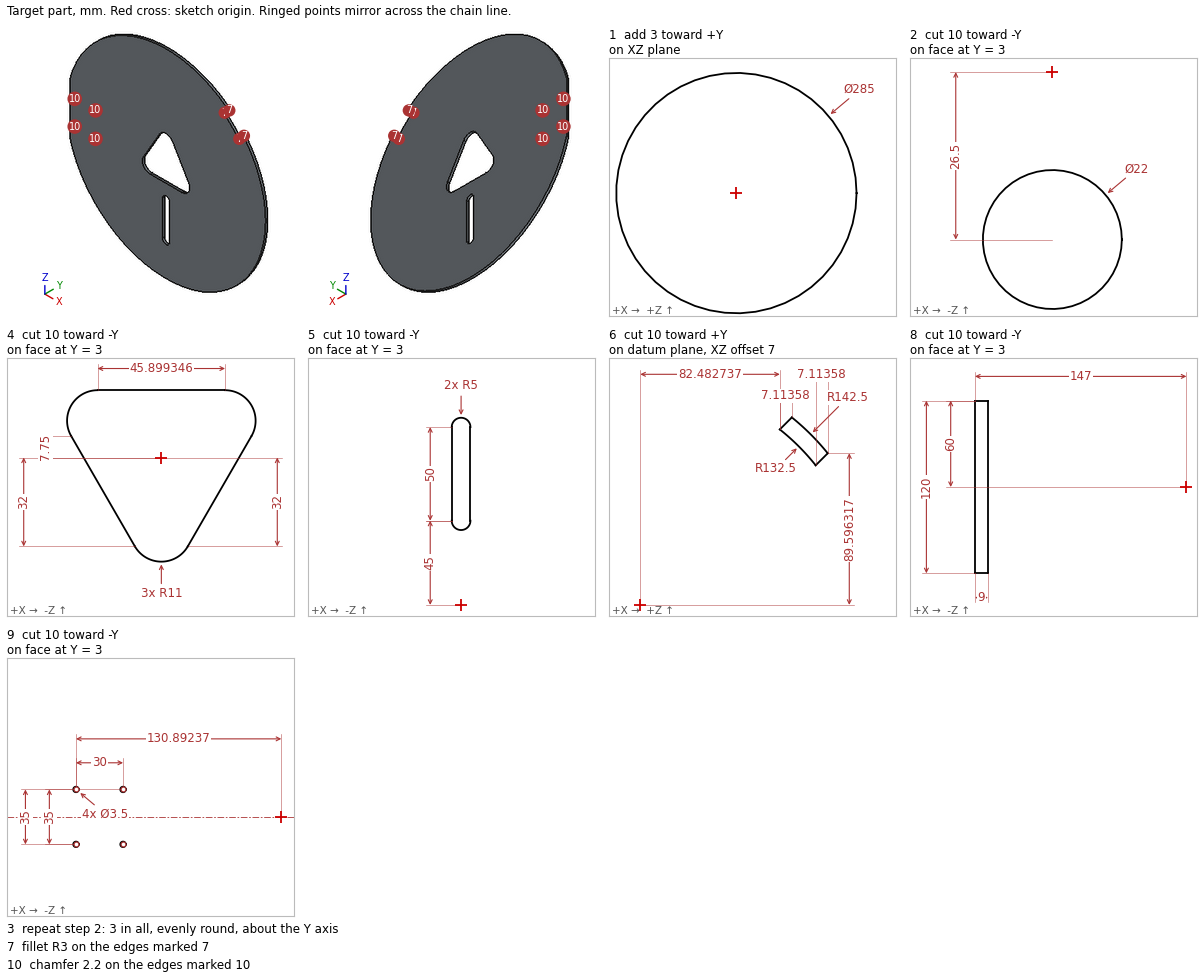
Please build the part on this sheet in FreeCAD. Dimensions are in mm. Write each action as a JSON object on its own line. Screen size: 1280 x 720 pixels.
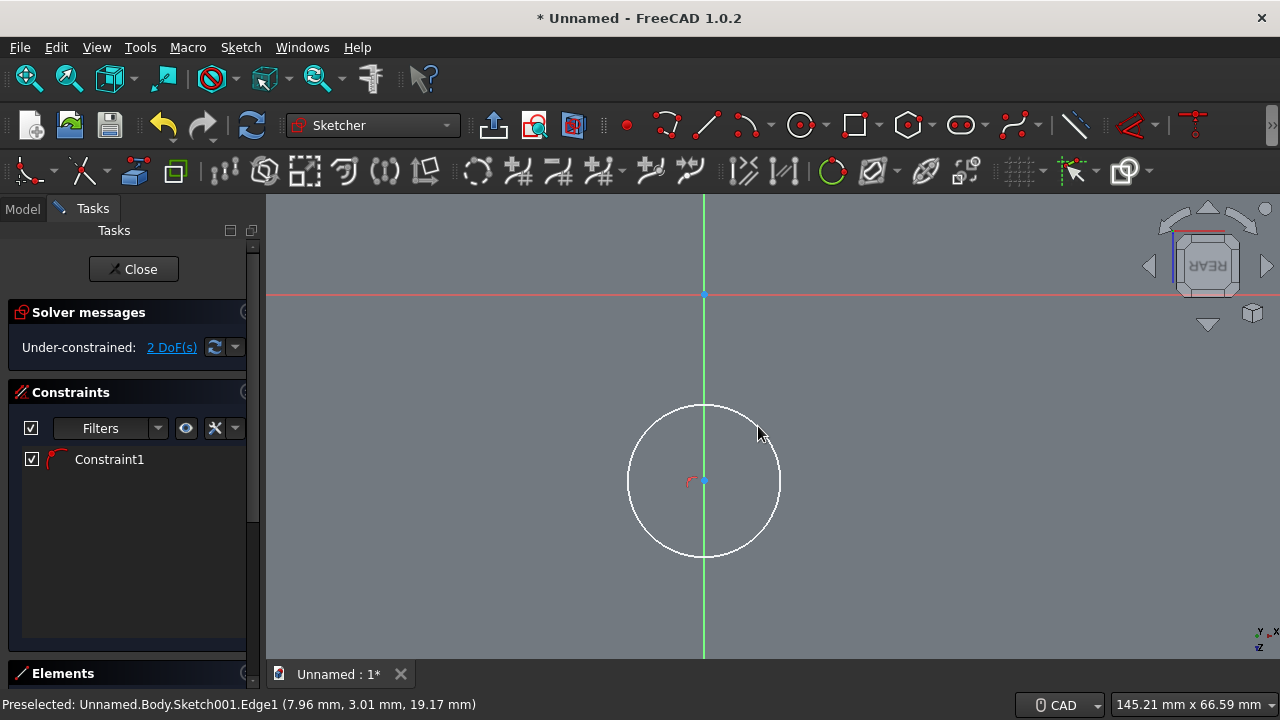
{"action": "left_click", "coordinate": [758, 427]}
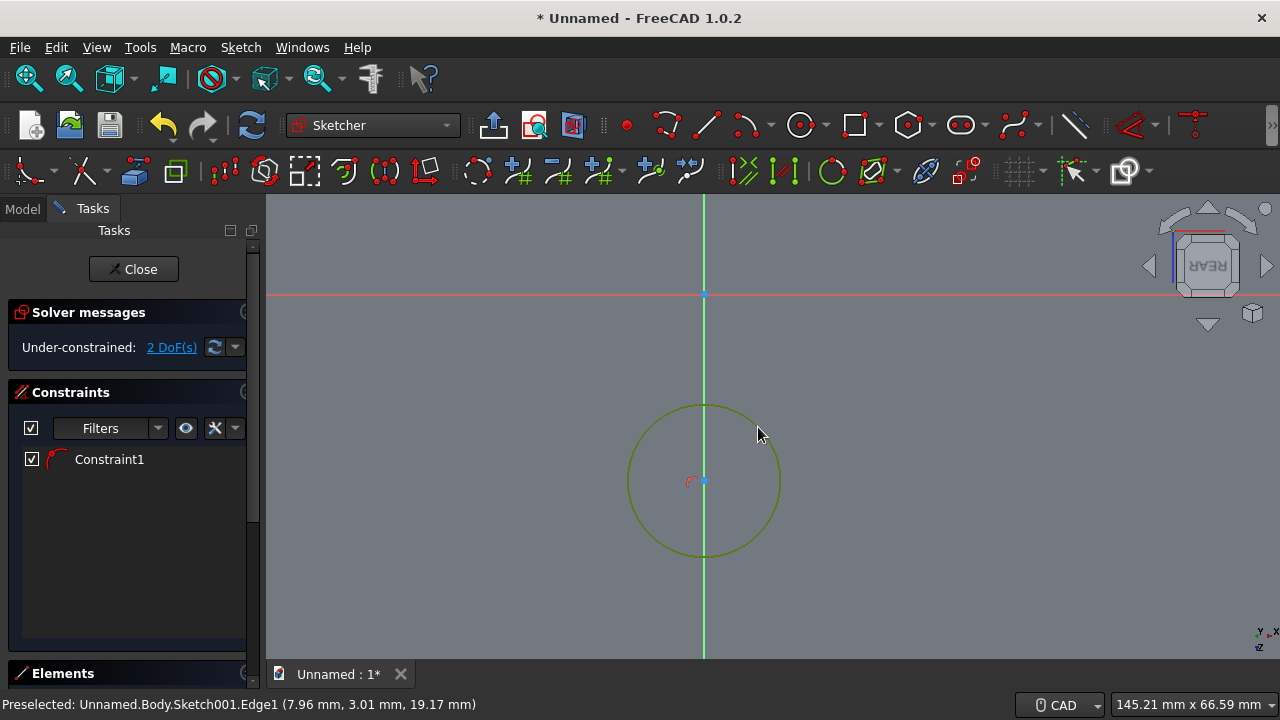
{"action": "key", "text": "k o"}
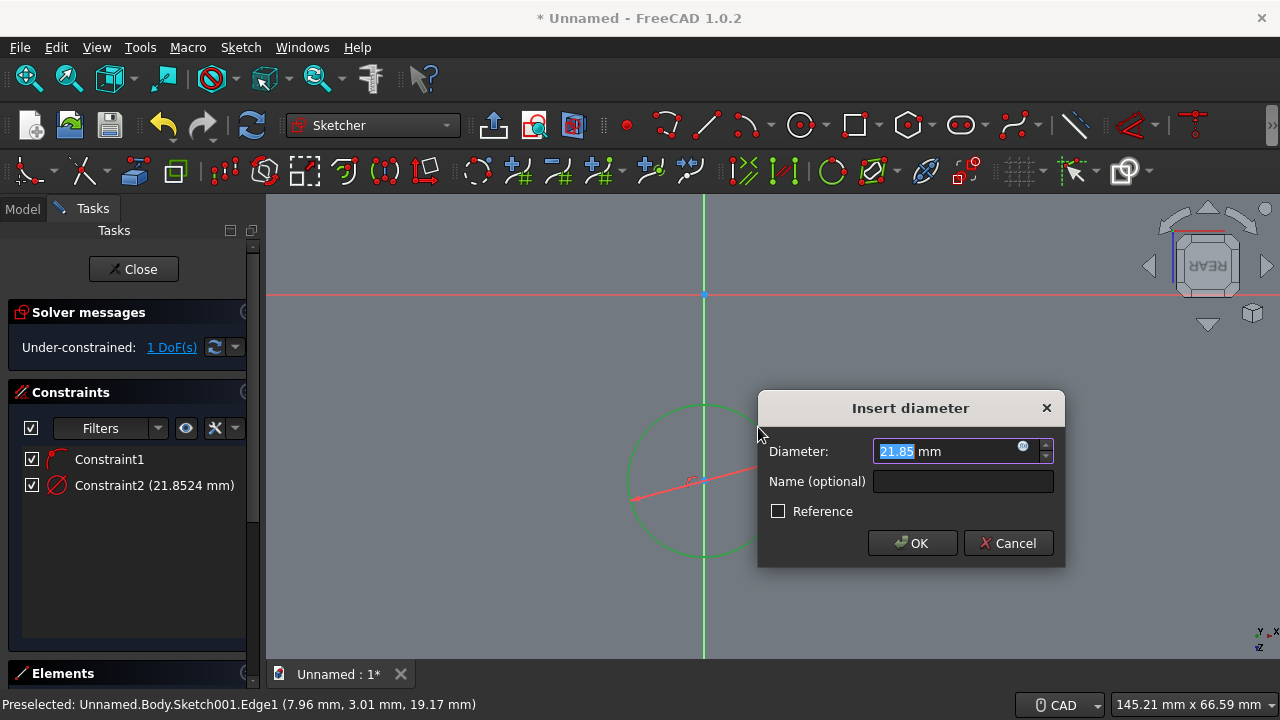
{"action": "type", "text": "22"}
{"action": "key", "text": "Return"}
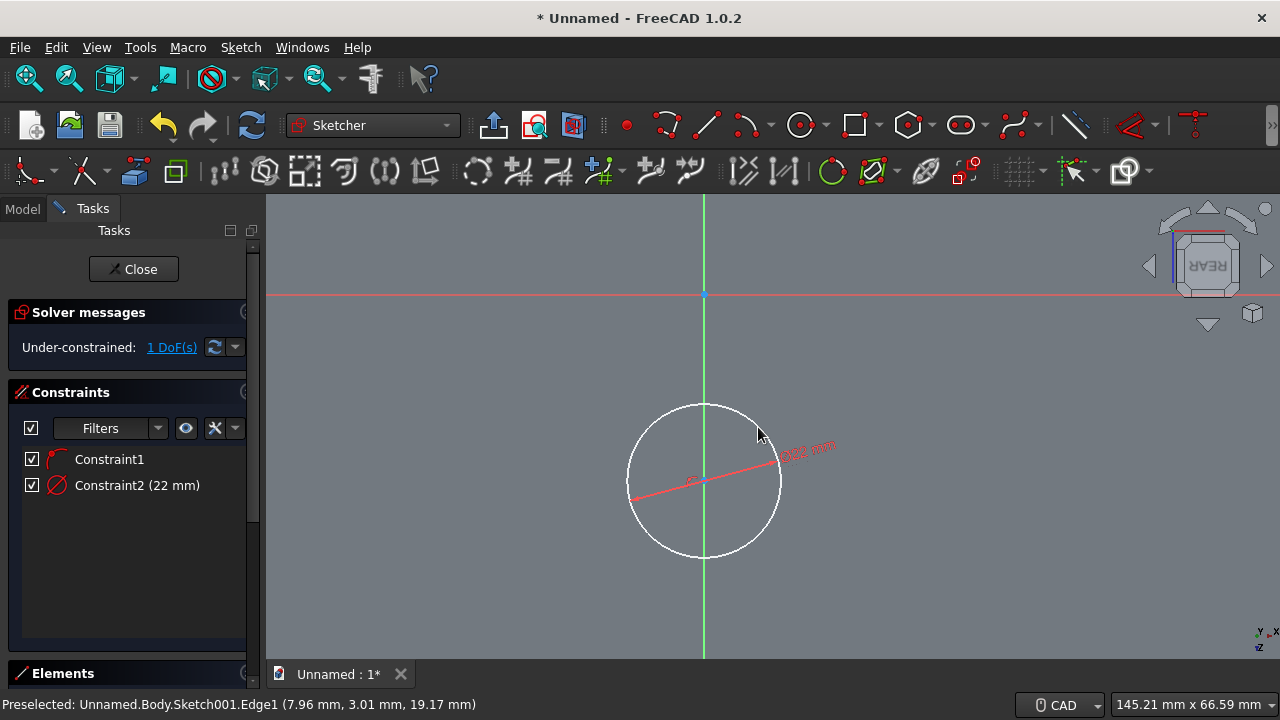
{"action": "left_click", "coordinate": [704, 481]}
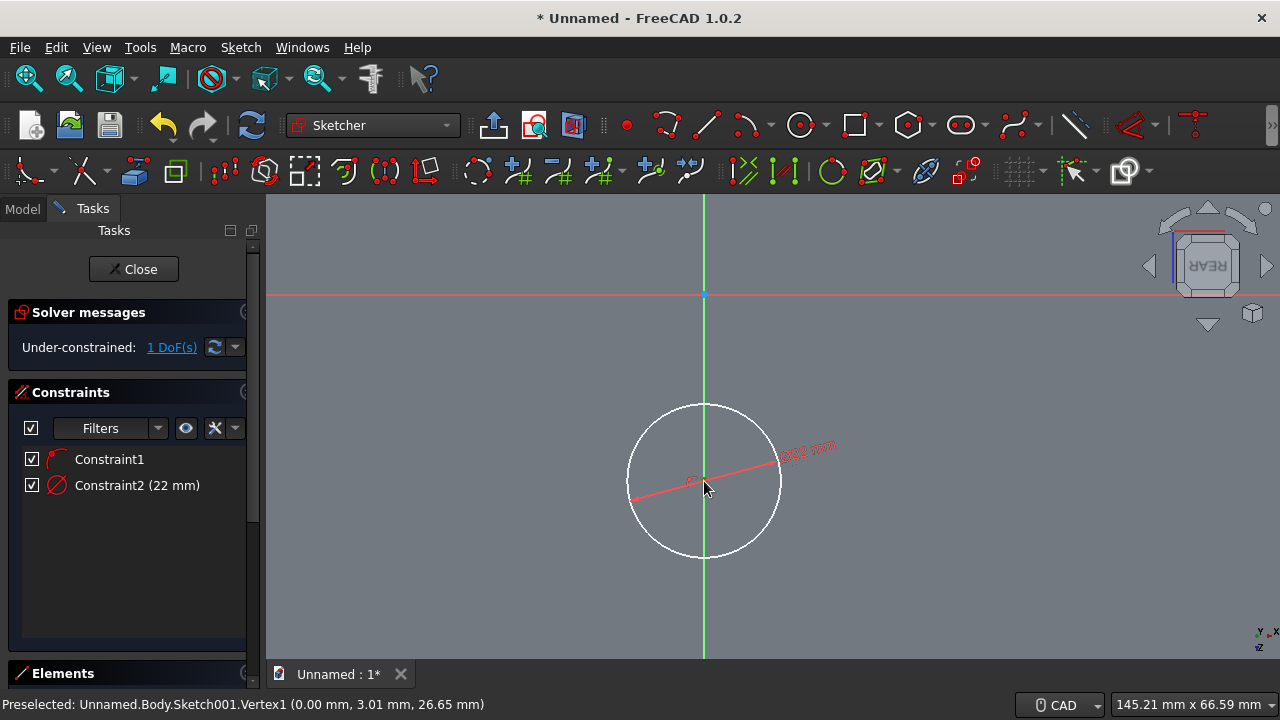
{"action": "left_click", "coordinate": [1158, 126]}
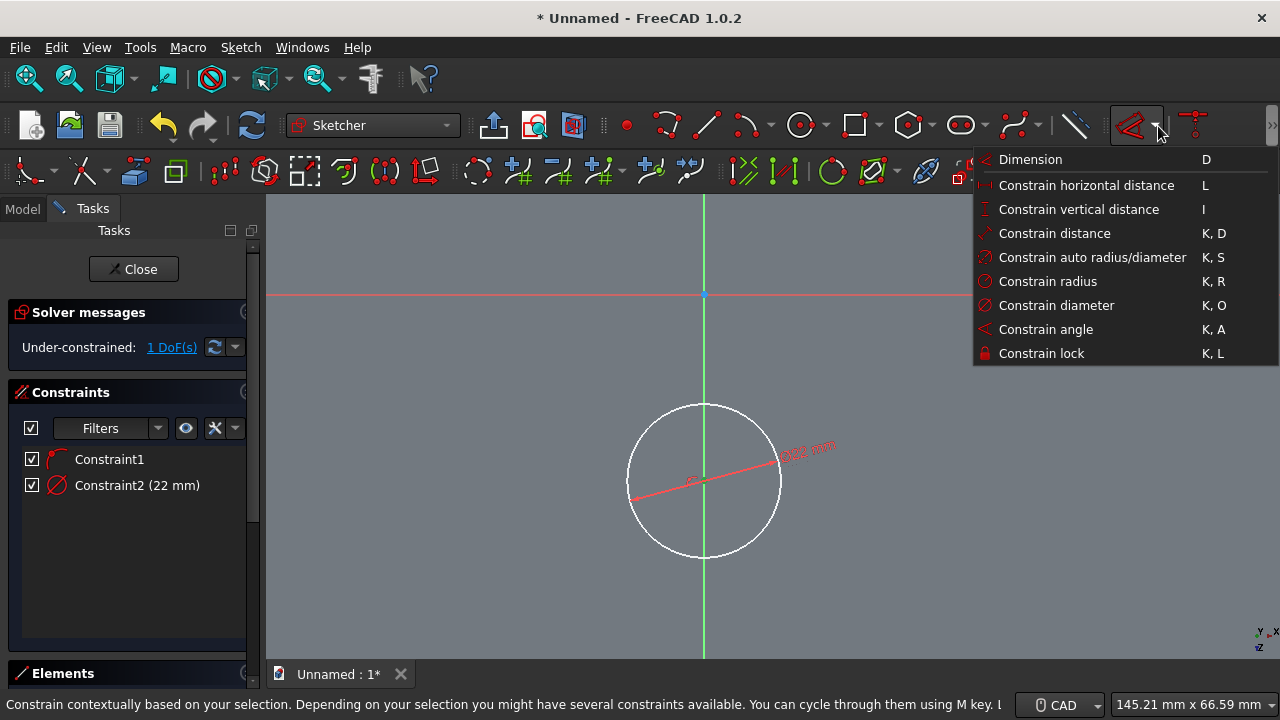
{"action": "left_click", "coordinate": [1126, 209]}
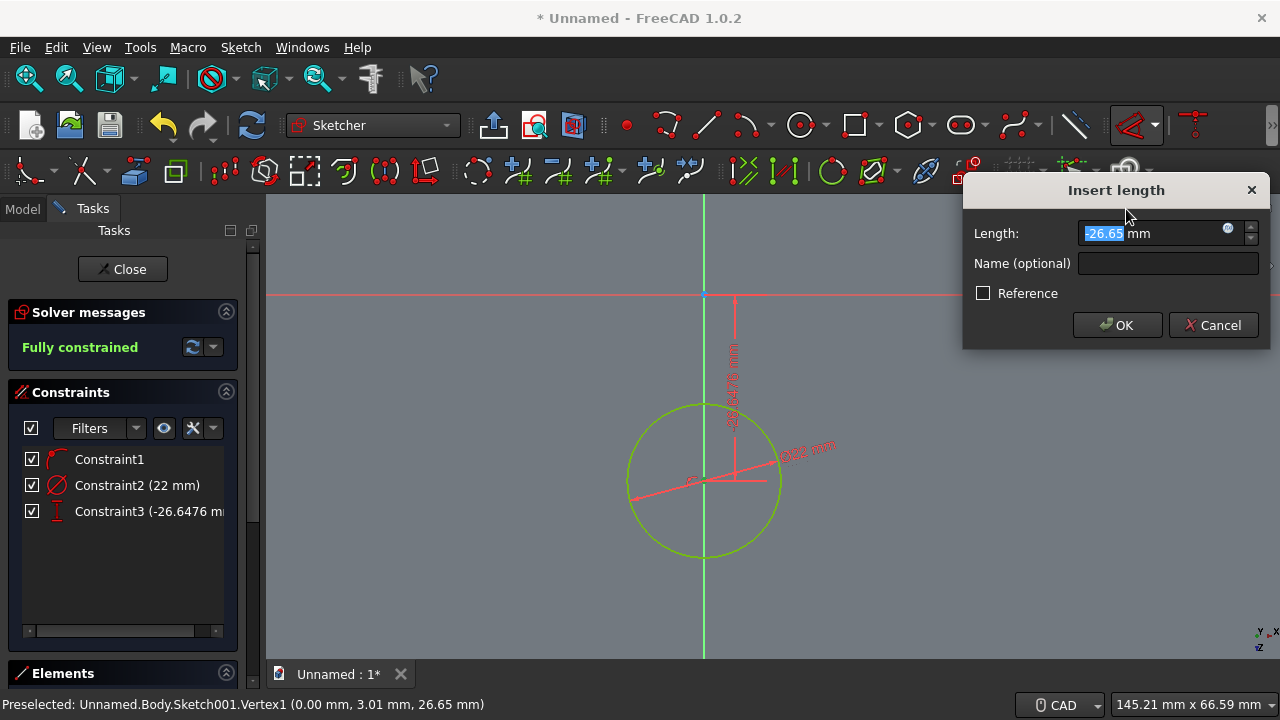
{"action": "type", "text": "-26.5"}
{"action": "key", "text": "Return"}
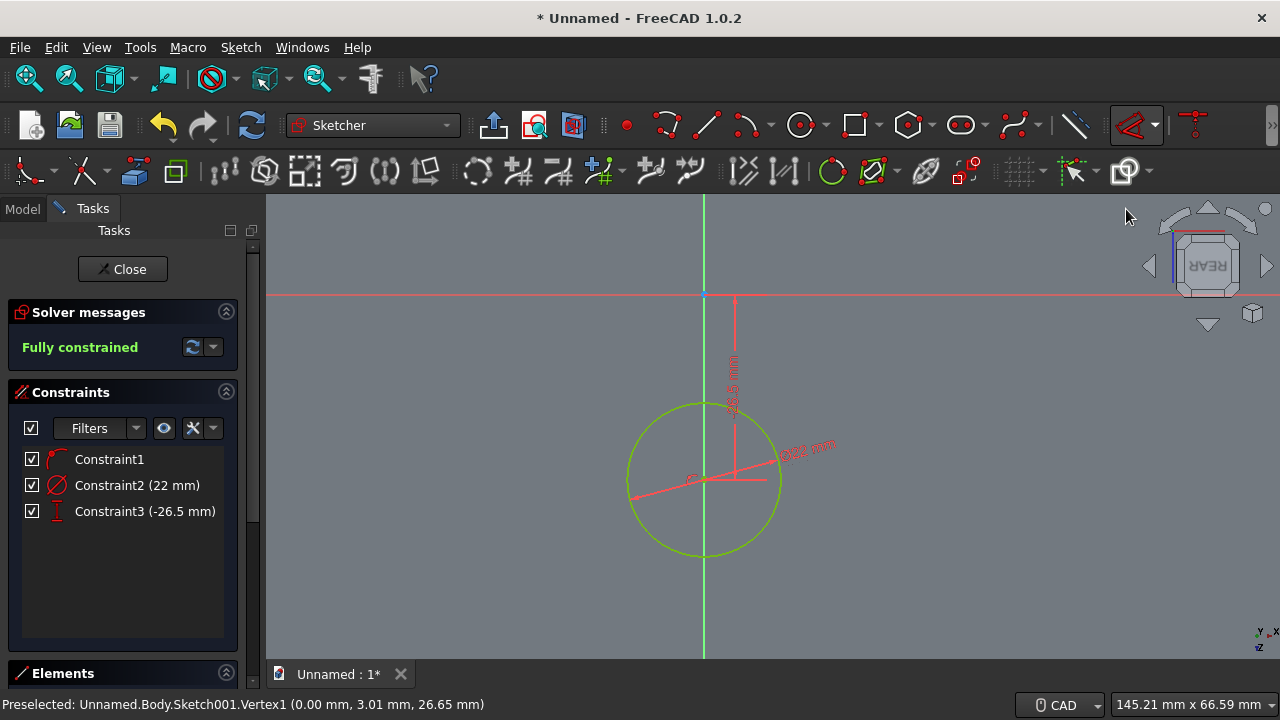
{"action": "left_click", "coordinate": [123, 269]}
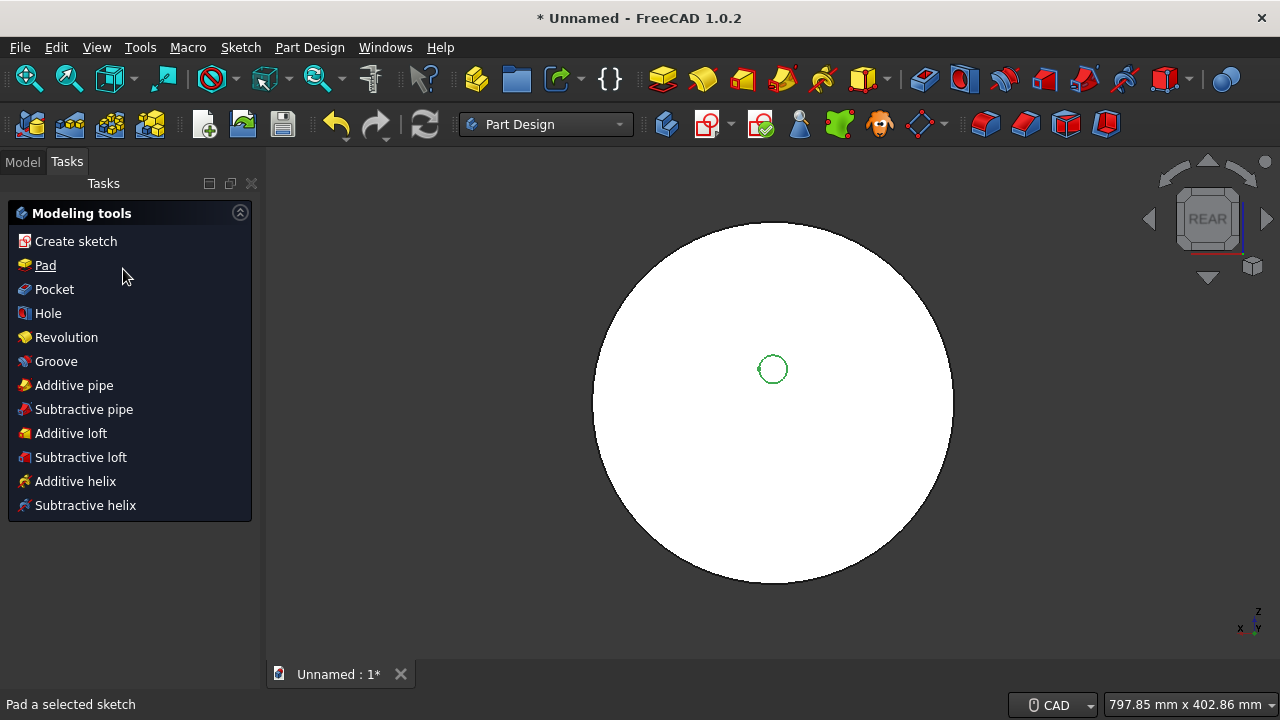
{"action": "left_click", "coordinate": [926, 80]}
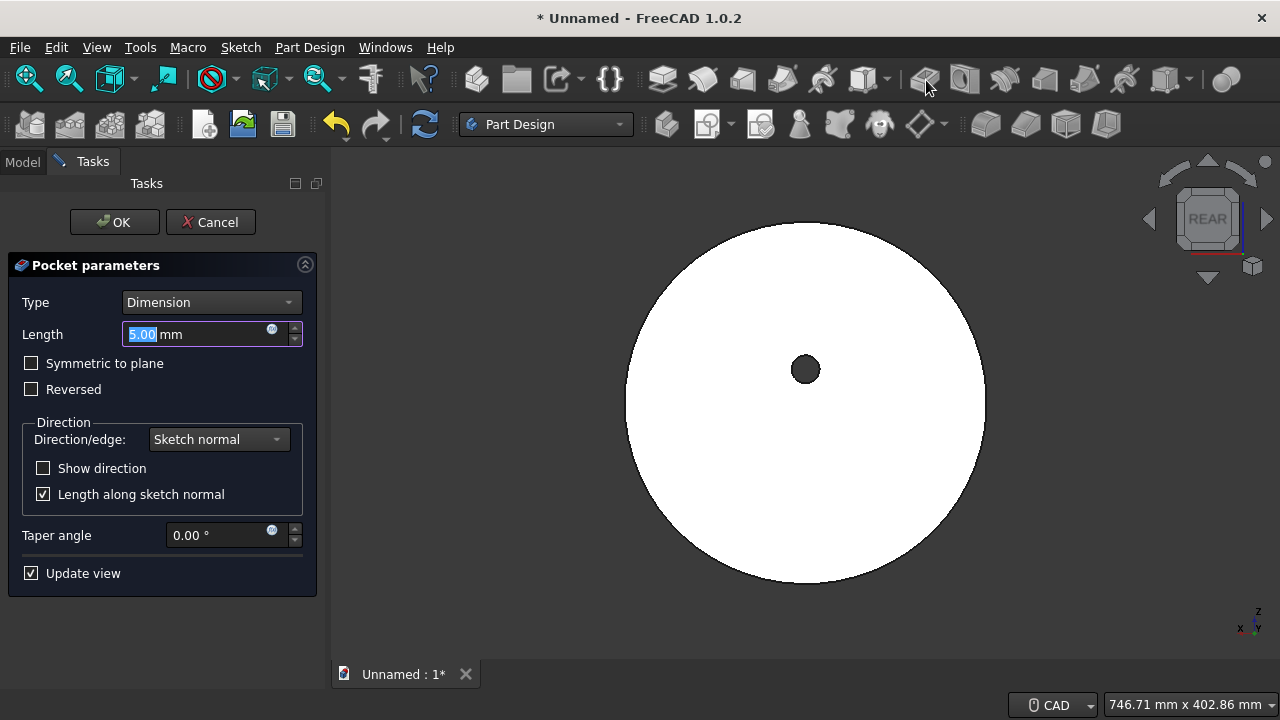
{"action": "type", "text": "10"}
{"action": "key", "text": "Tab"}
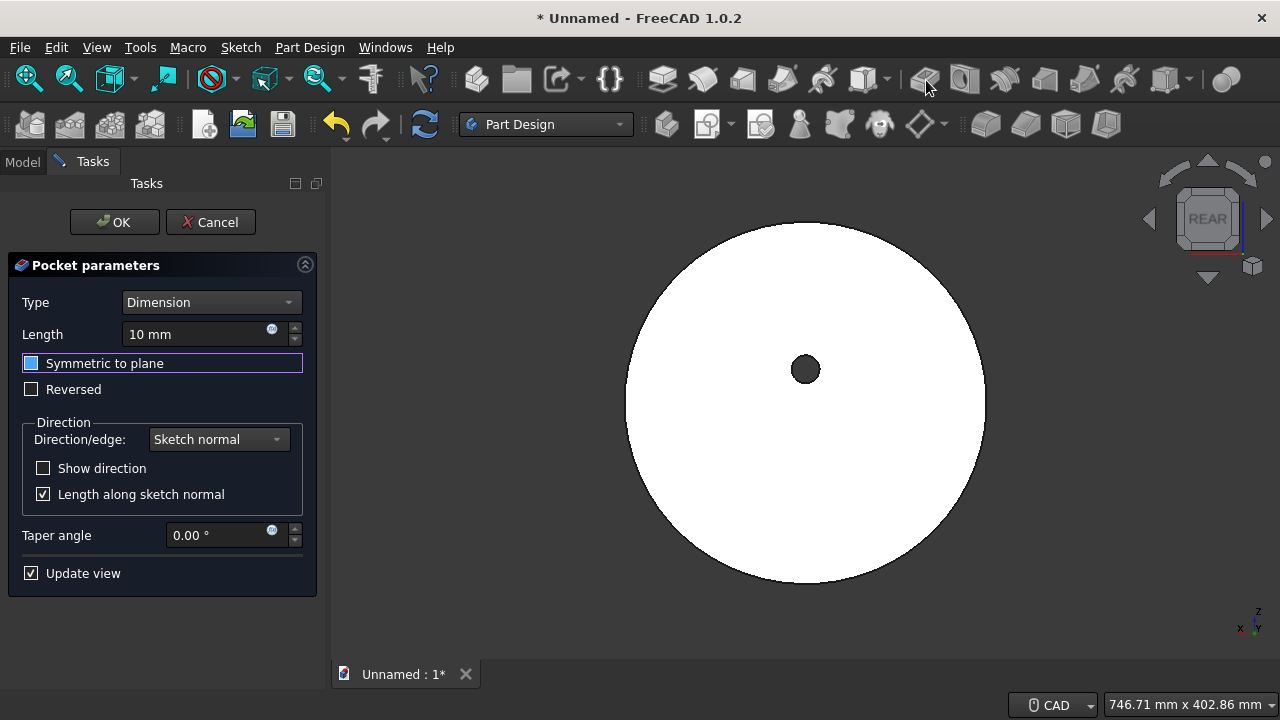
{"action": "left_click", "coordinate": [115, 222]}